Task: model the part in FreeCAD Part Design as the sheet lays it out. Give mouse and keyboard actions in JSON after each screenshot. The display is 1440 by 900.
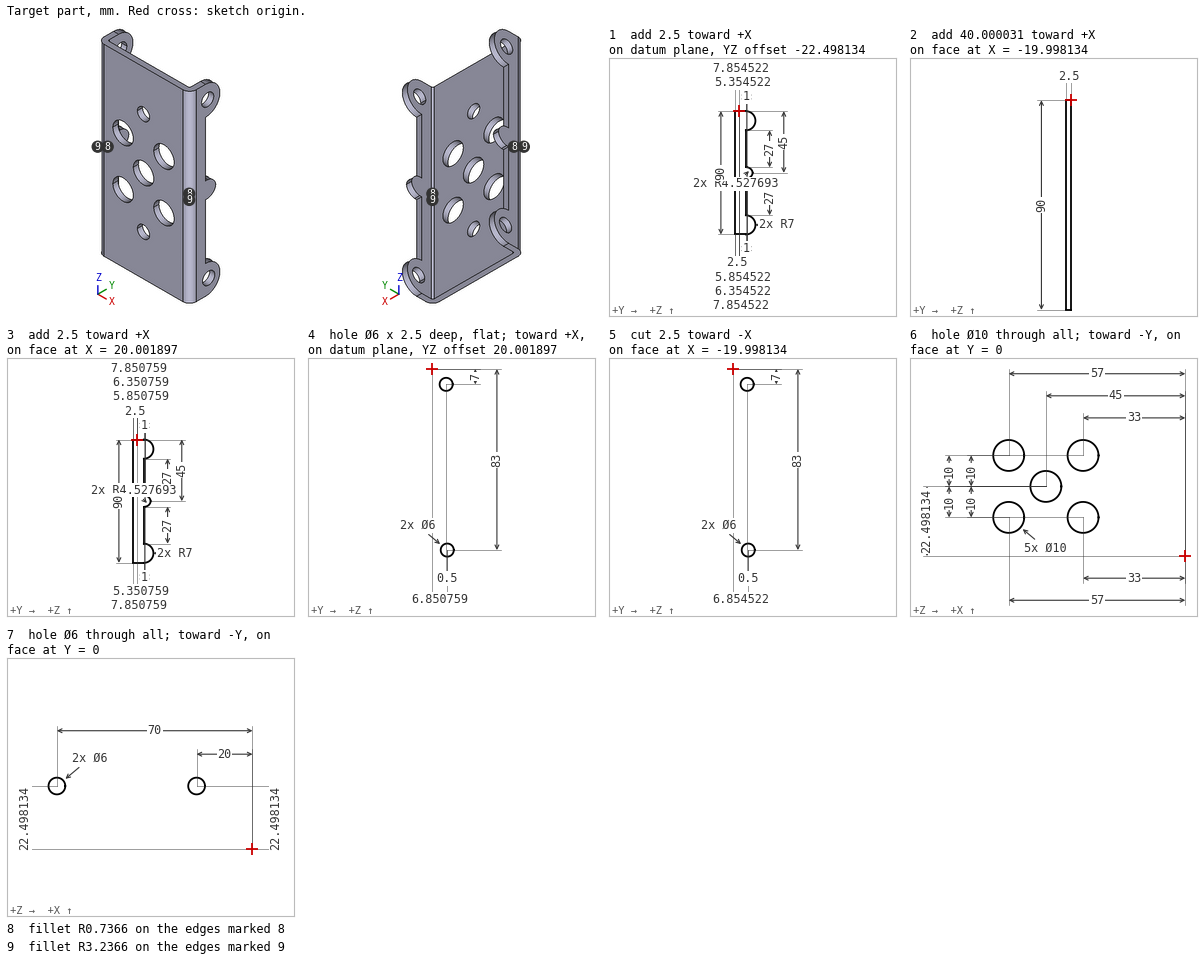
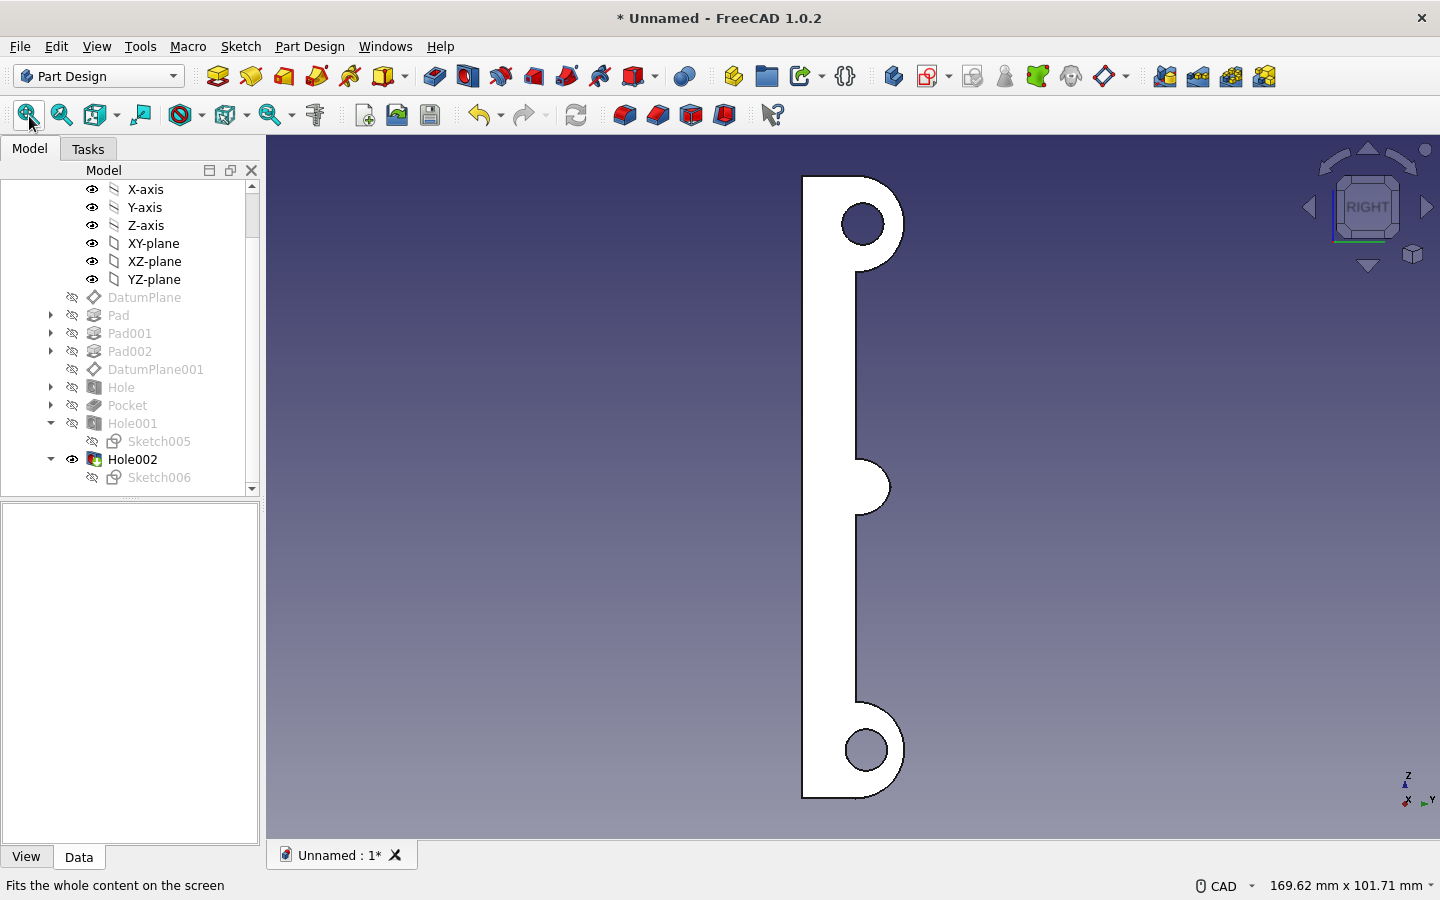
{"action": "key", "text": "5"}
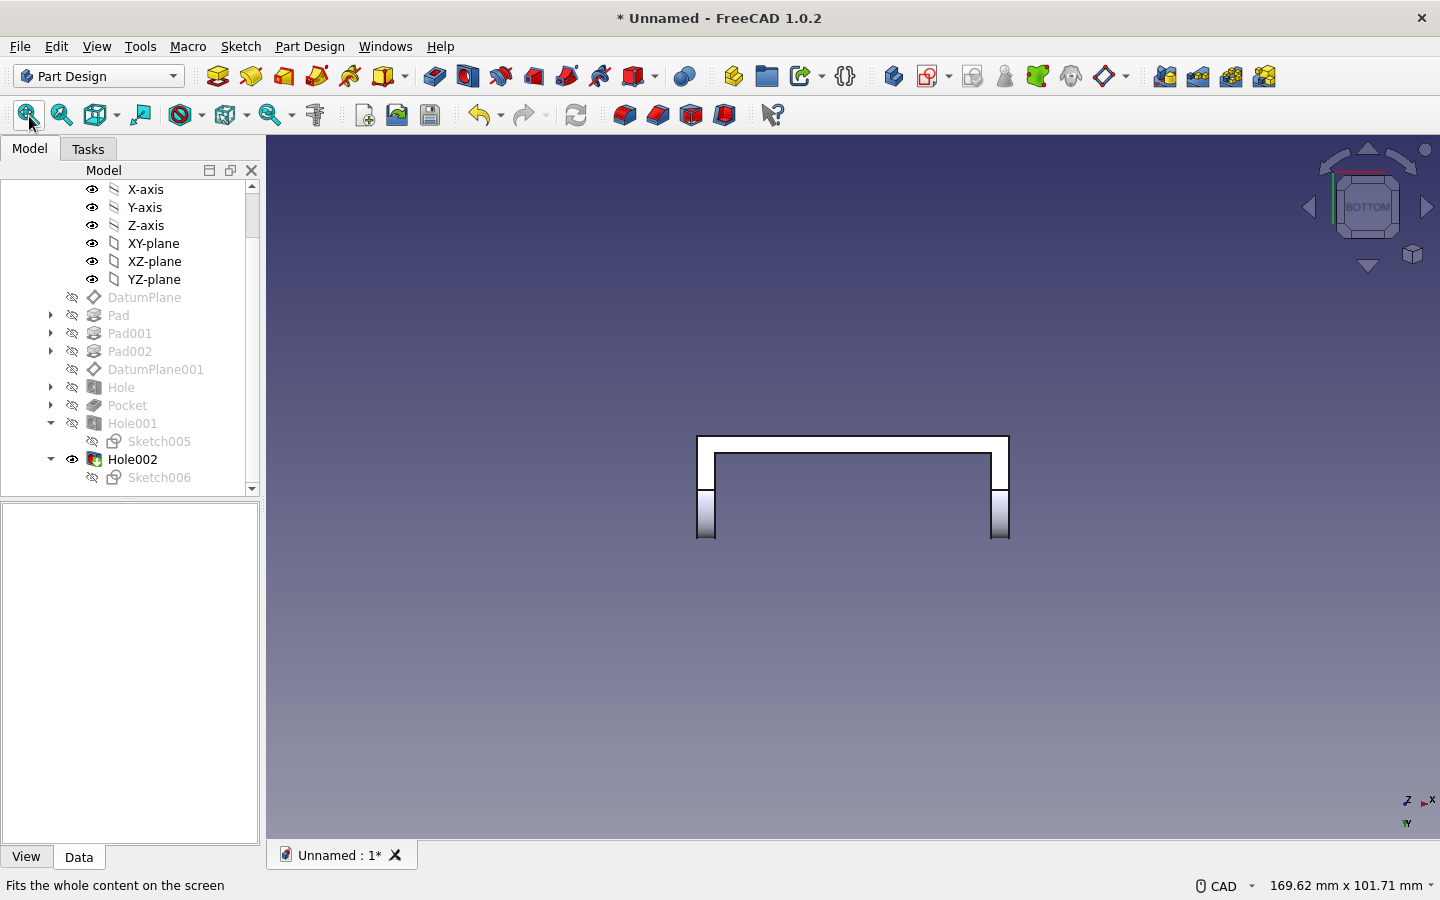
{"action": "left_click", "coordinate": [29, 116]}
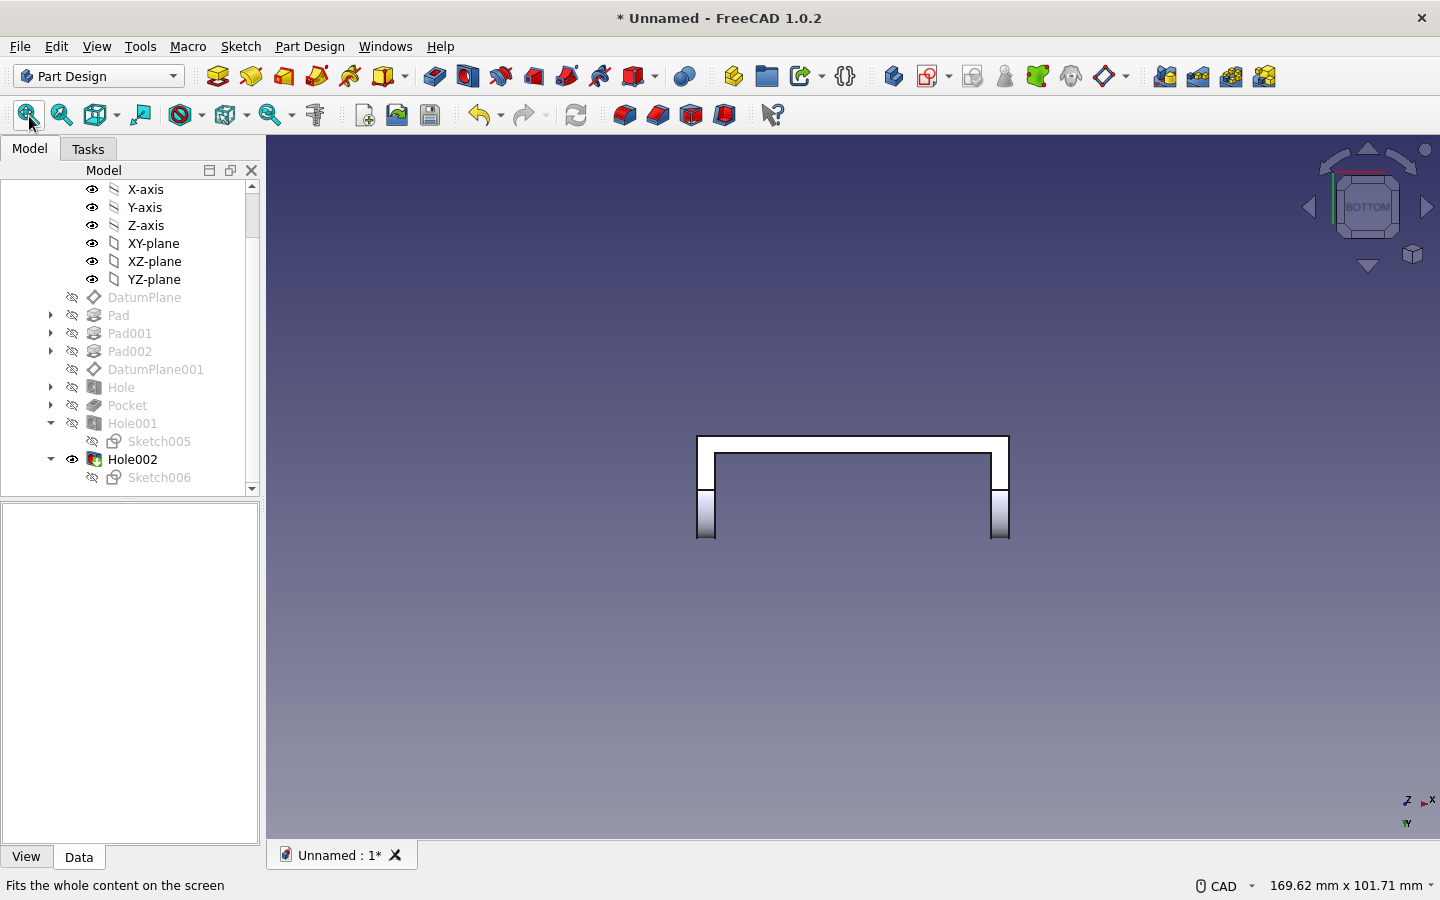
{"action": "key", "text": "4"}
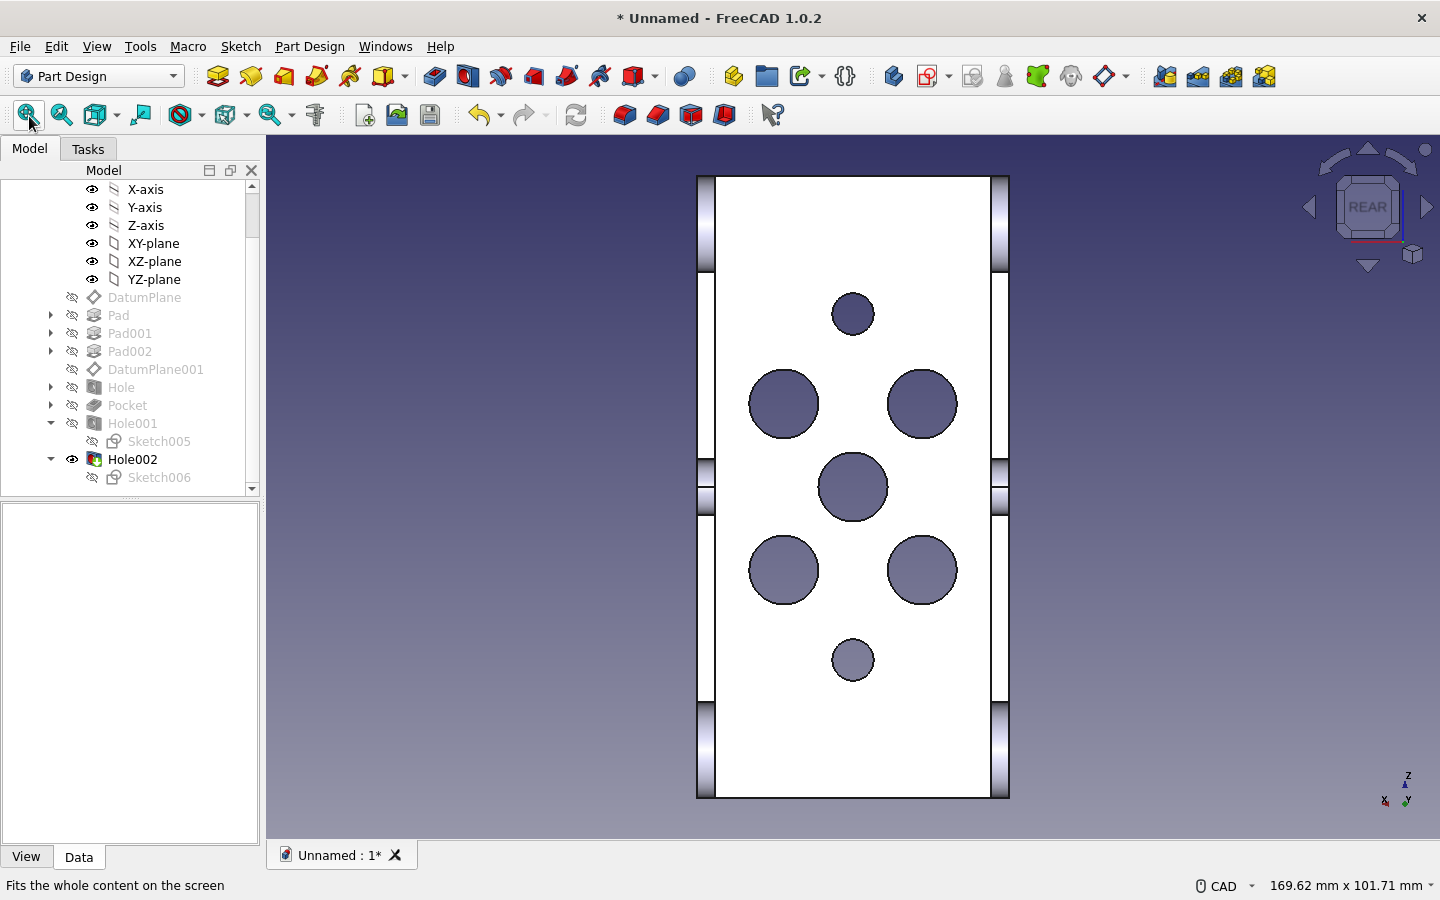
{"action": "key", "text": "6"}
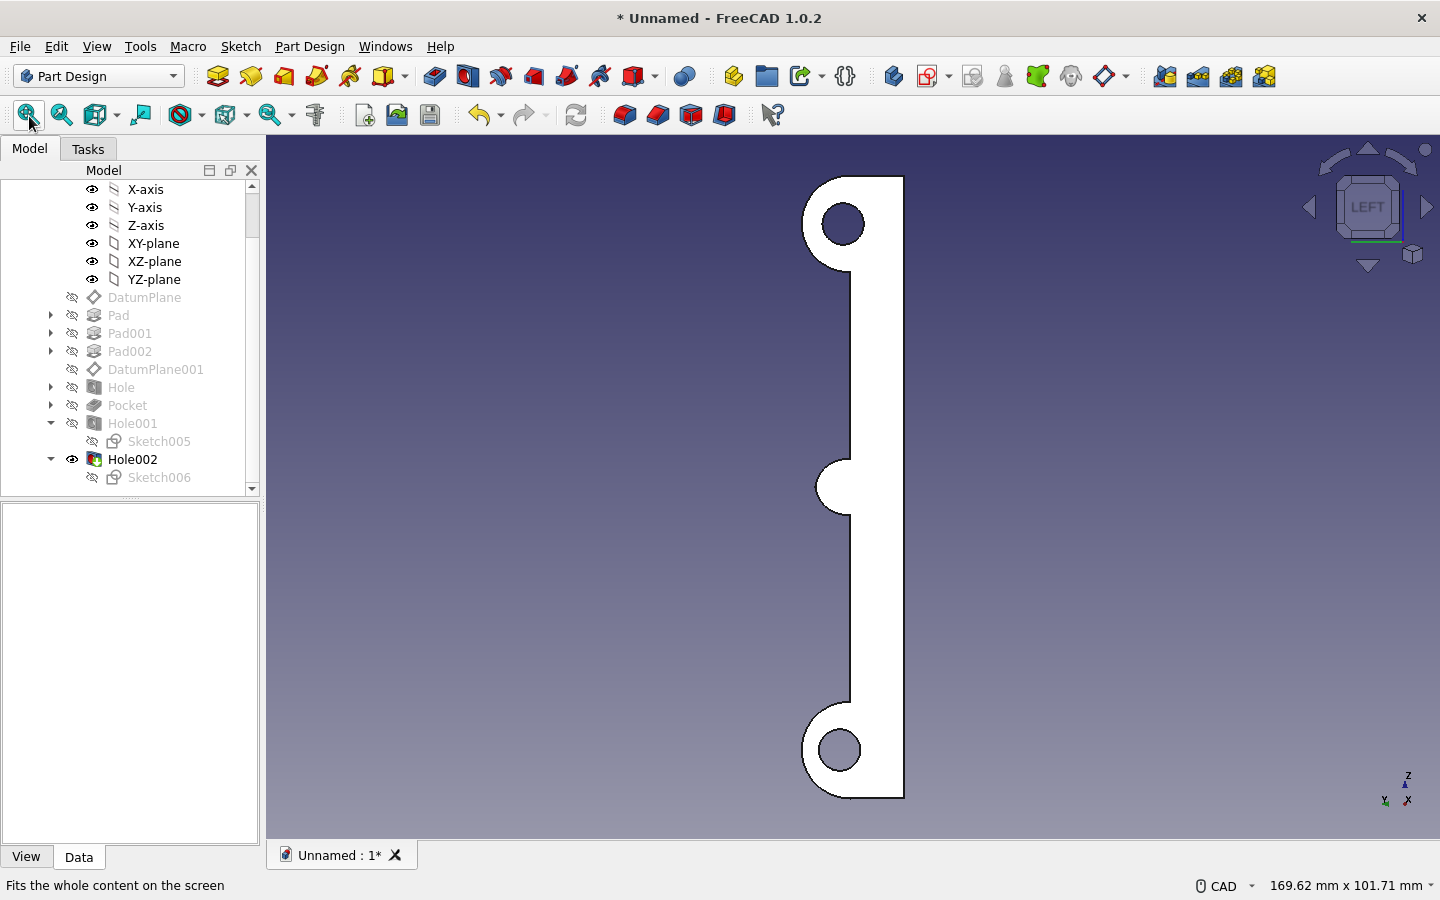
{"action": "key", "text": "v 3"}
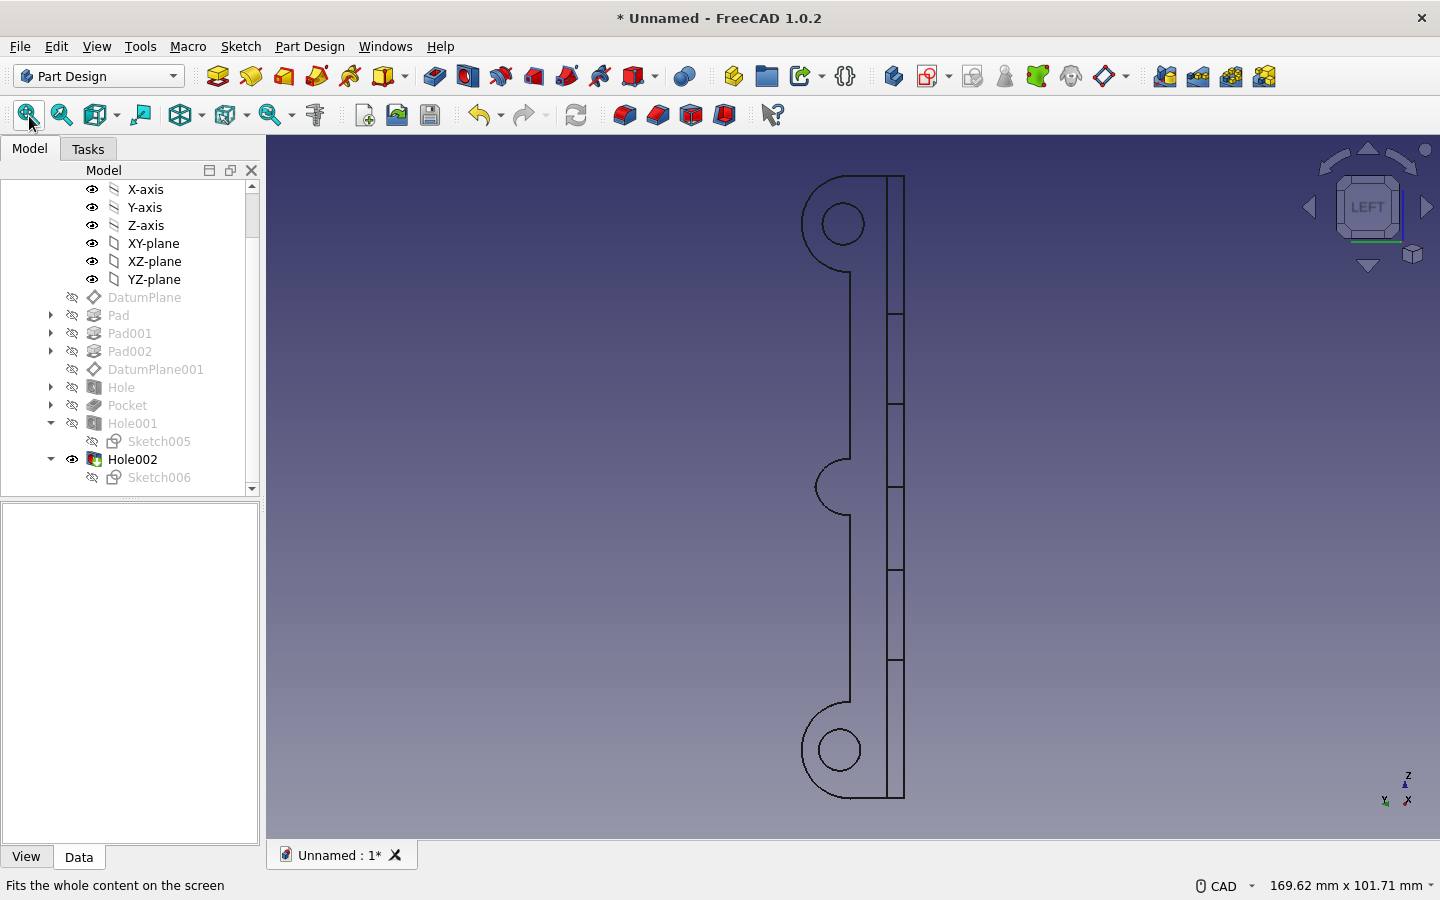
{"action": "key", "text": "0"}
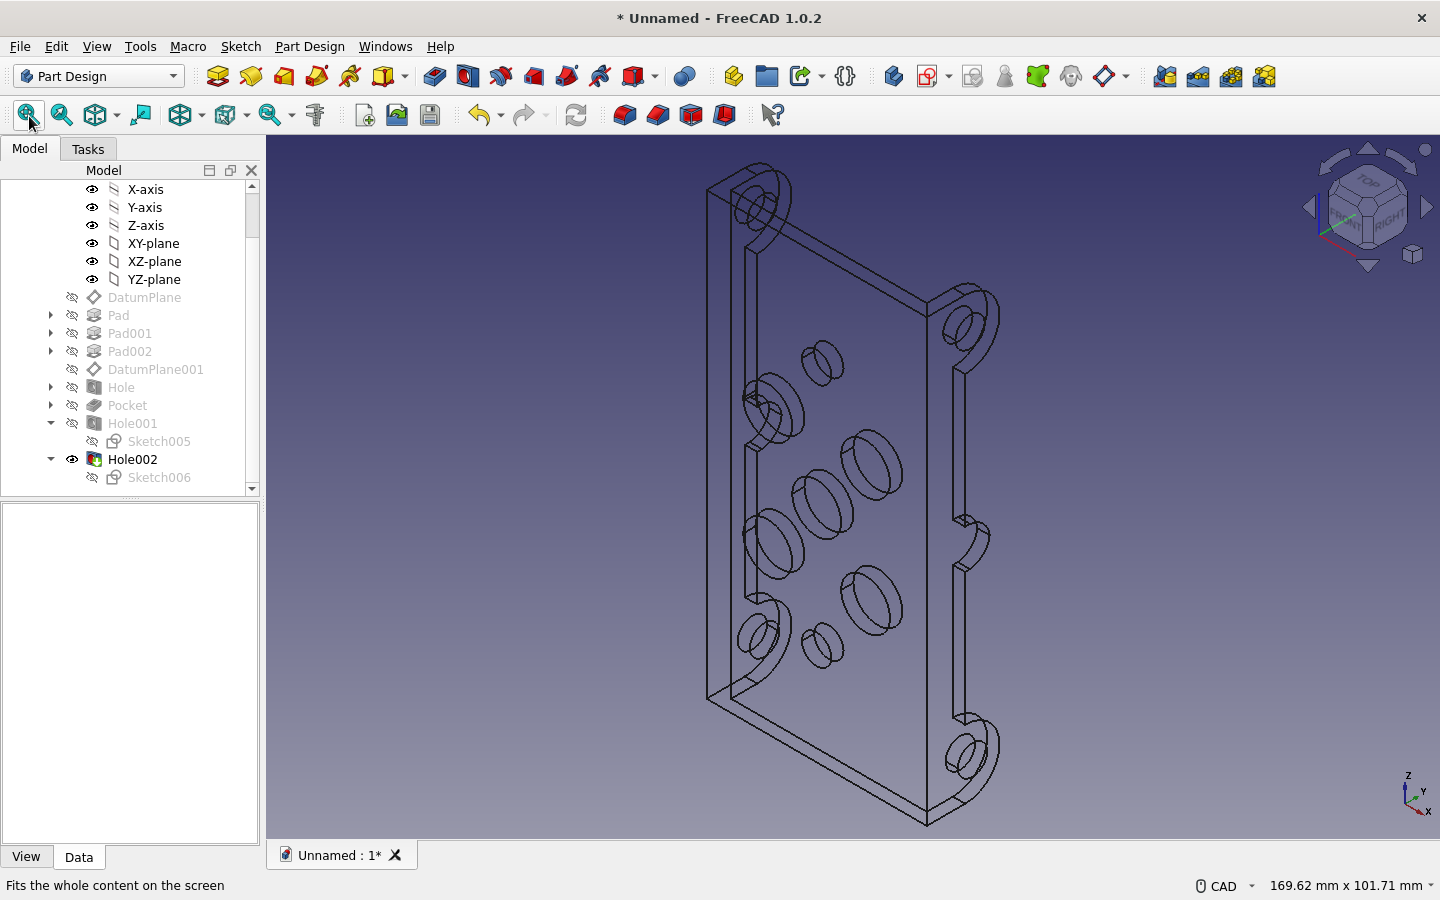
{"action": "left_click", "coordinate": [731, 443]}